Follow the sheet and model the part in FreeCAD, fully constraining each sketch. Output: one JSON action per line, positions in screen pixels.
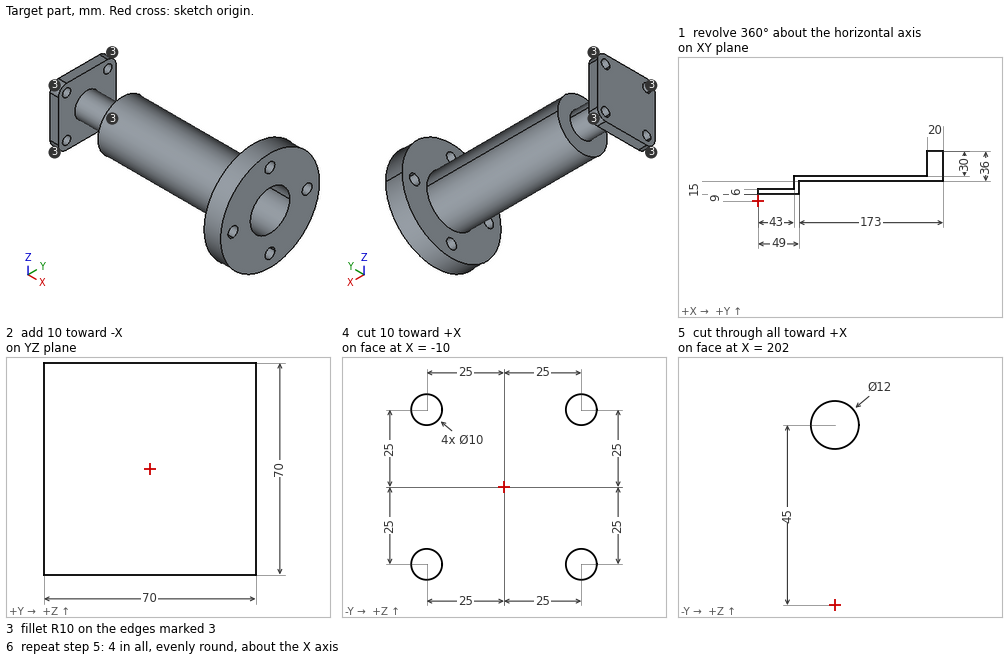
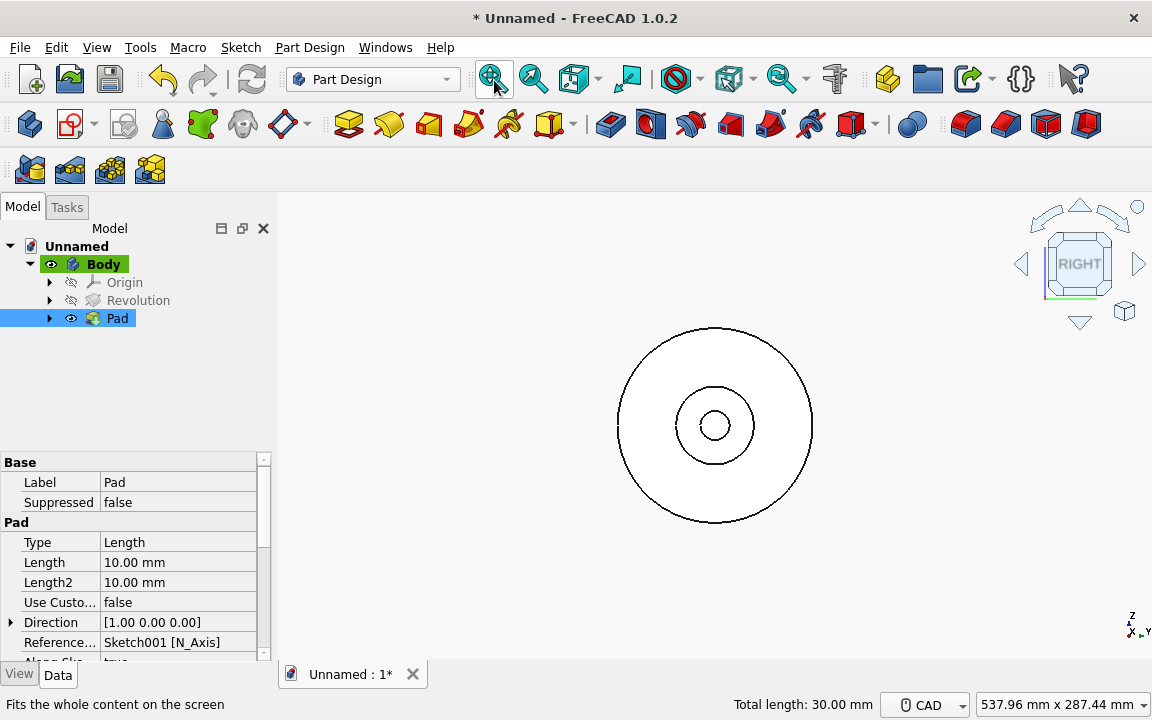
{"action": "left_click", "coordinate": [494, 80]}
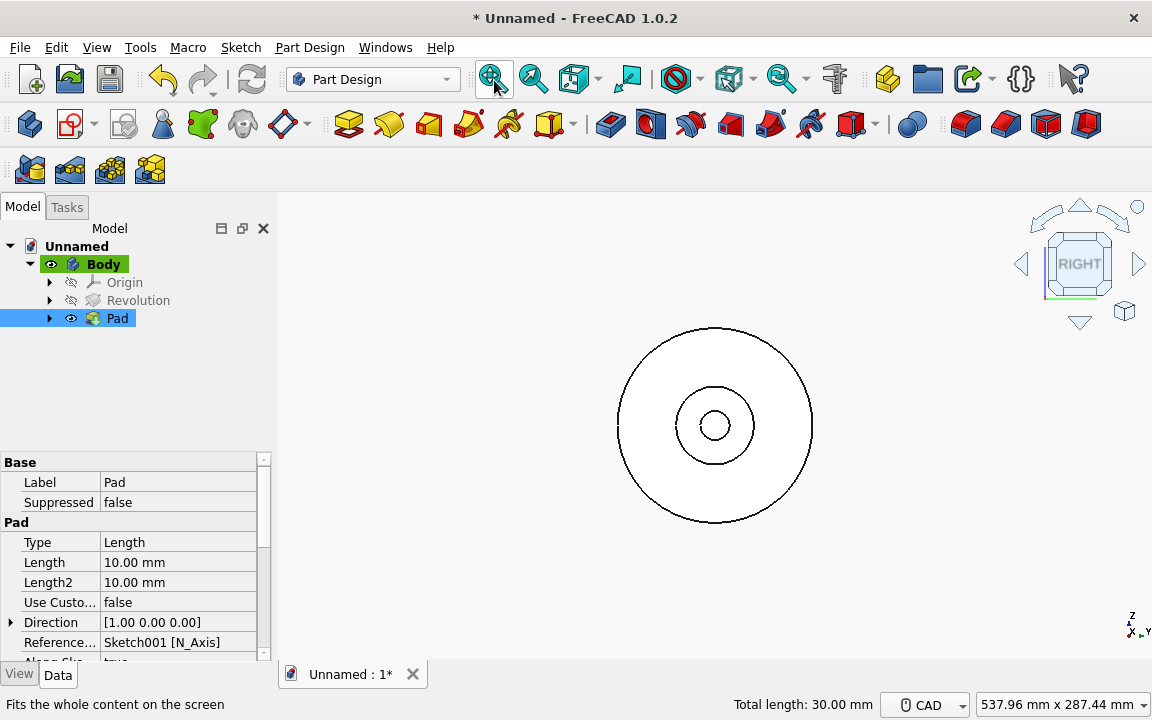
{"action": "scroll", "coordinate": [772, 481], "scroll_direction": "up", "scroll_amount": 5}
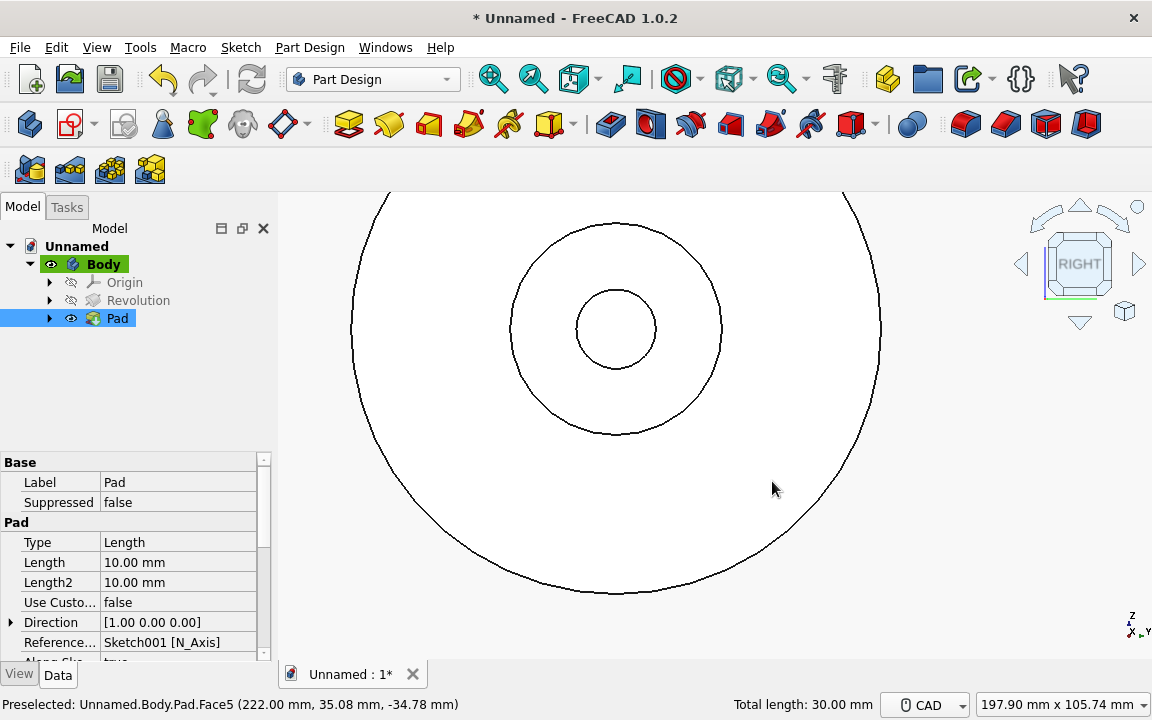
{"action": "left_click", "coordinate": [494, 80]}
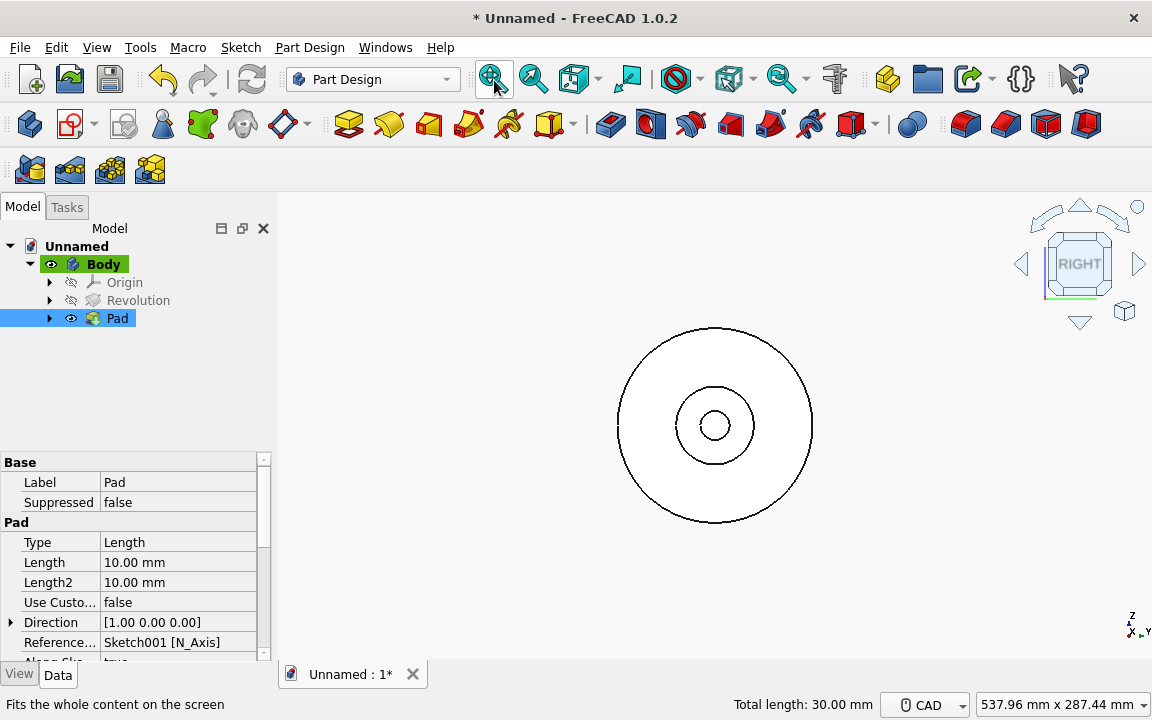
{"action": "key", "text": "5"}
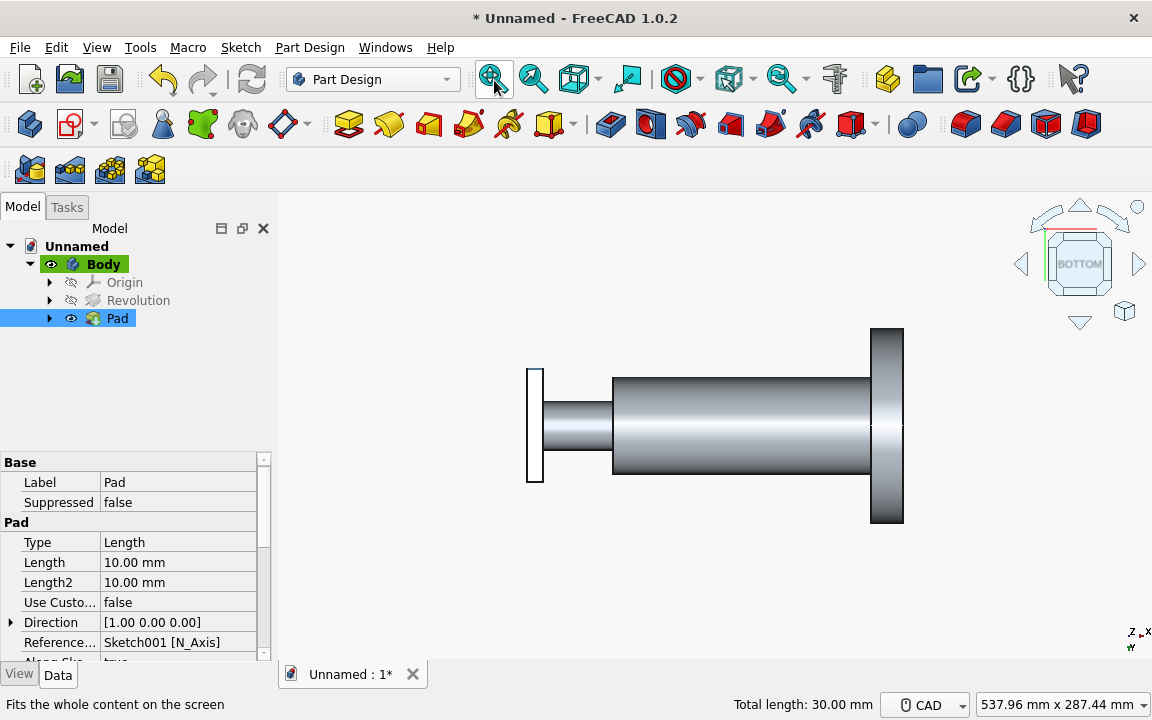
{"action": "key", "text": "v f"}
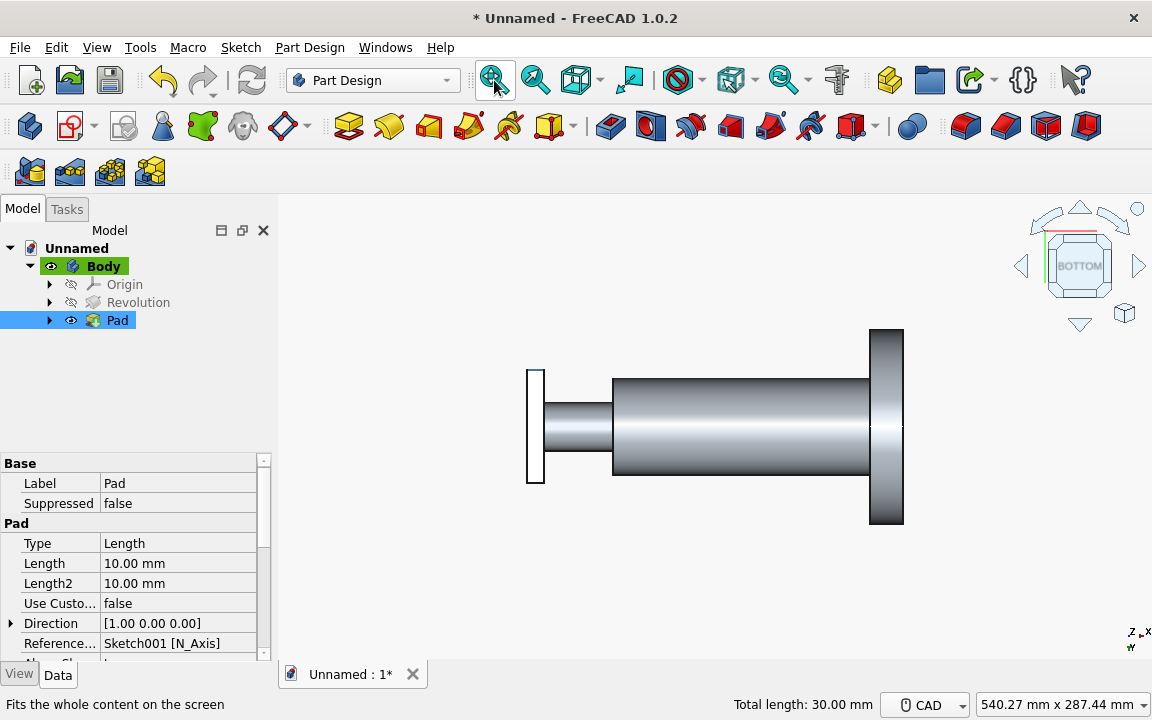
{"action": "left_click", "coordinate": [535, 482], "text": "ctrl"}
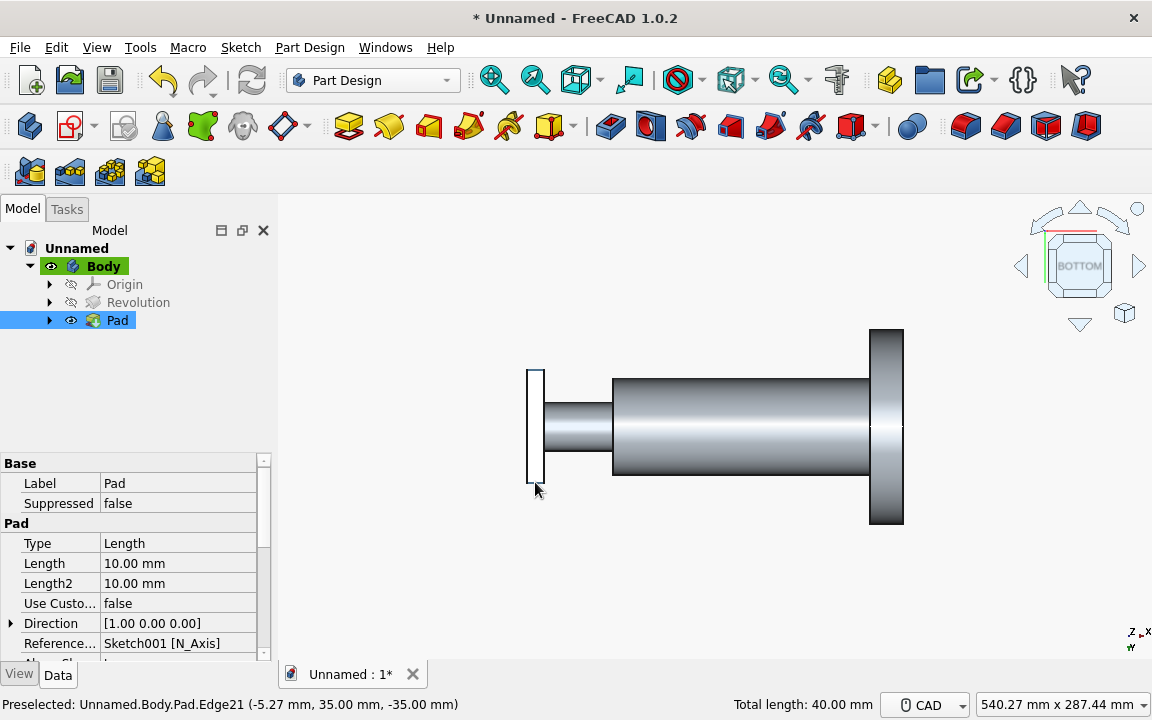
{"action": "left_click", "coordinate": [966, 126]}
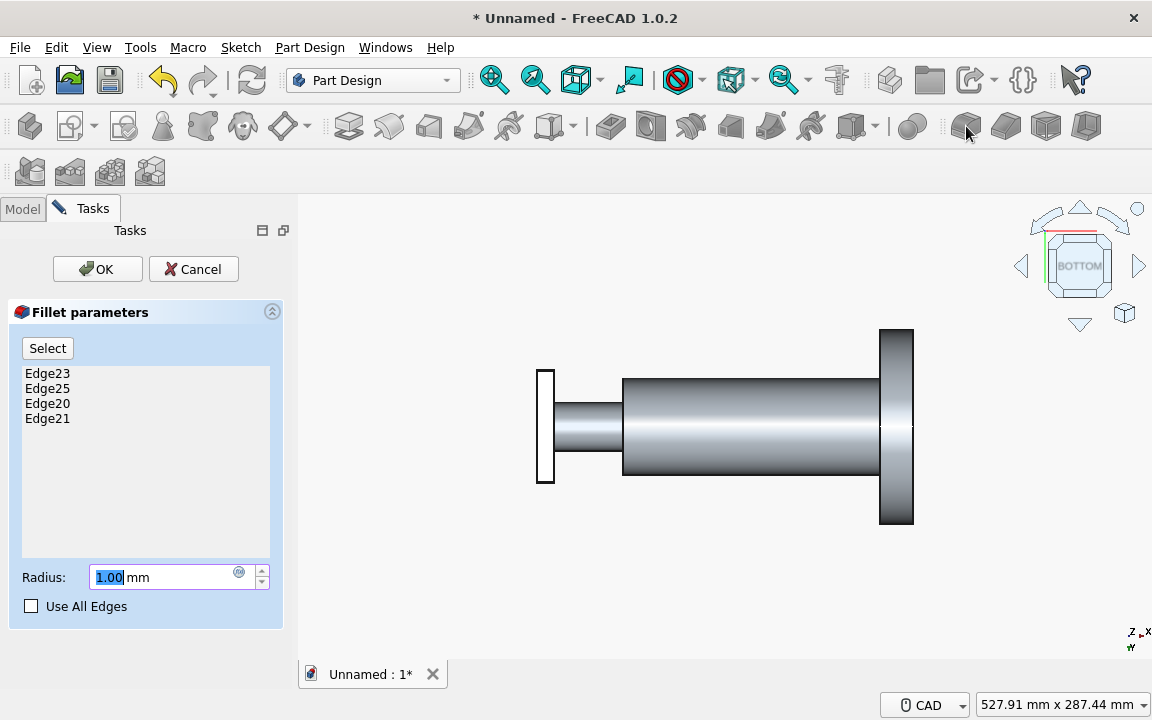
{"action": "type", "text": "10"}
{"action": "key", "text": "Tab"}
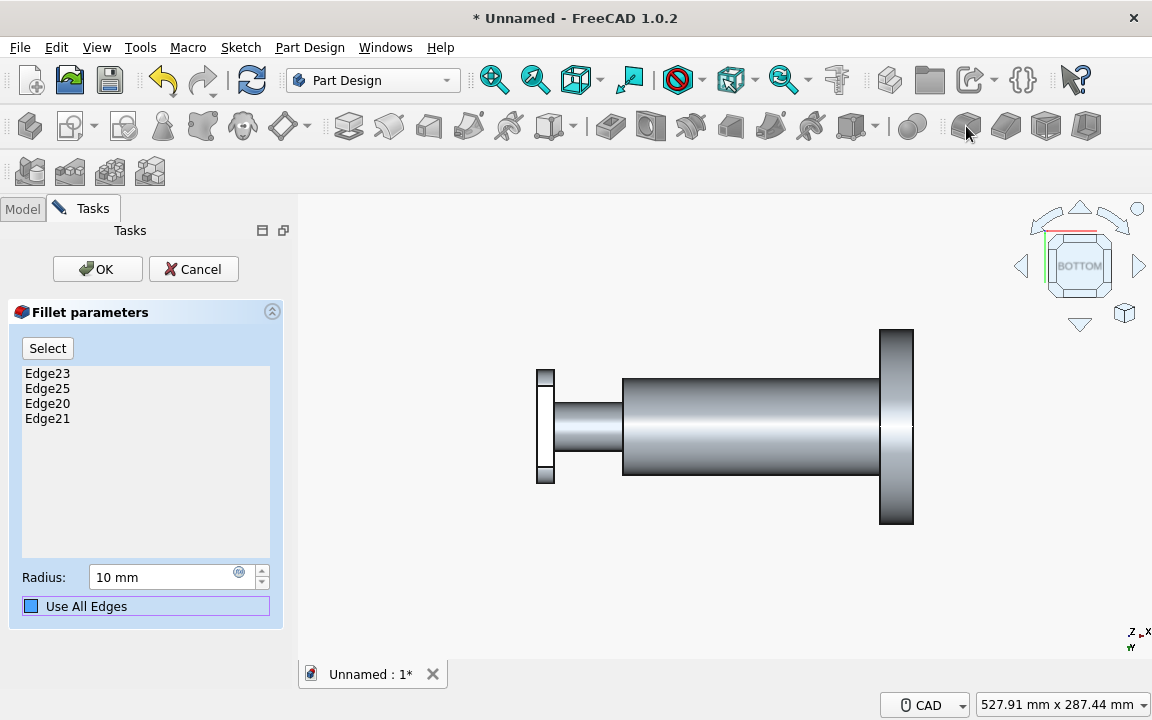
{"action": "left_click", "coordinate": [98, 269]}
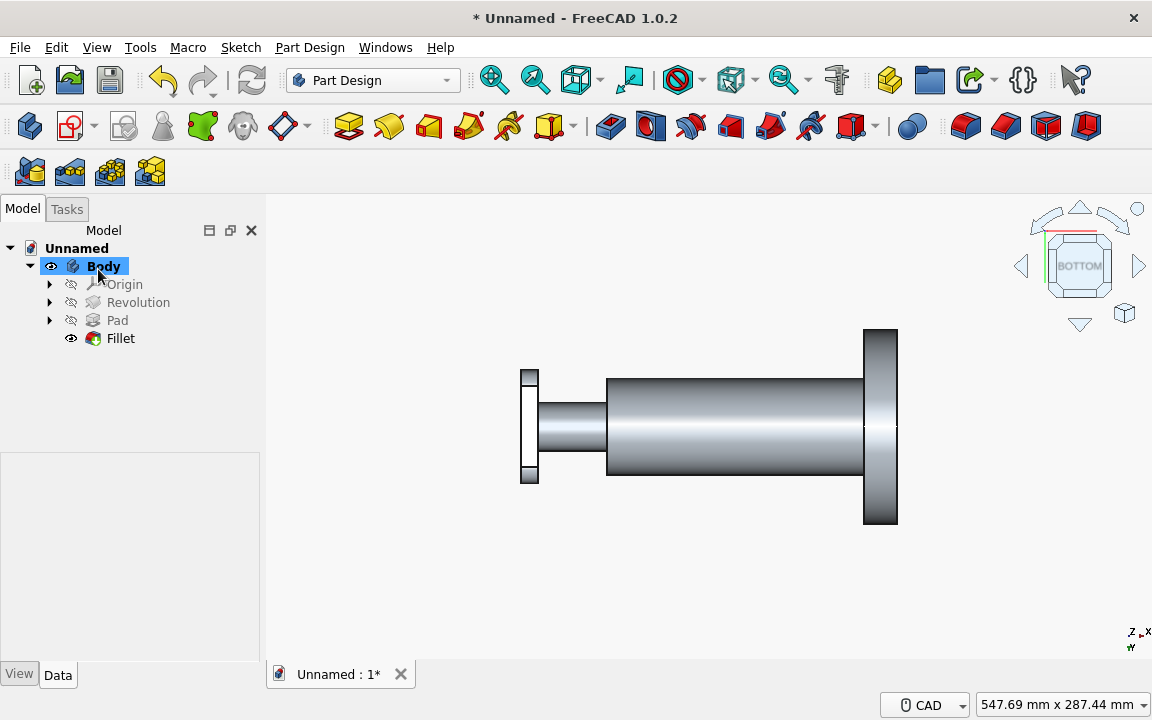
{"action": "left_click", "coordinate": [496, 80]}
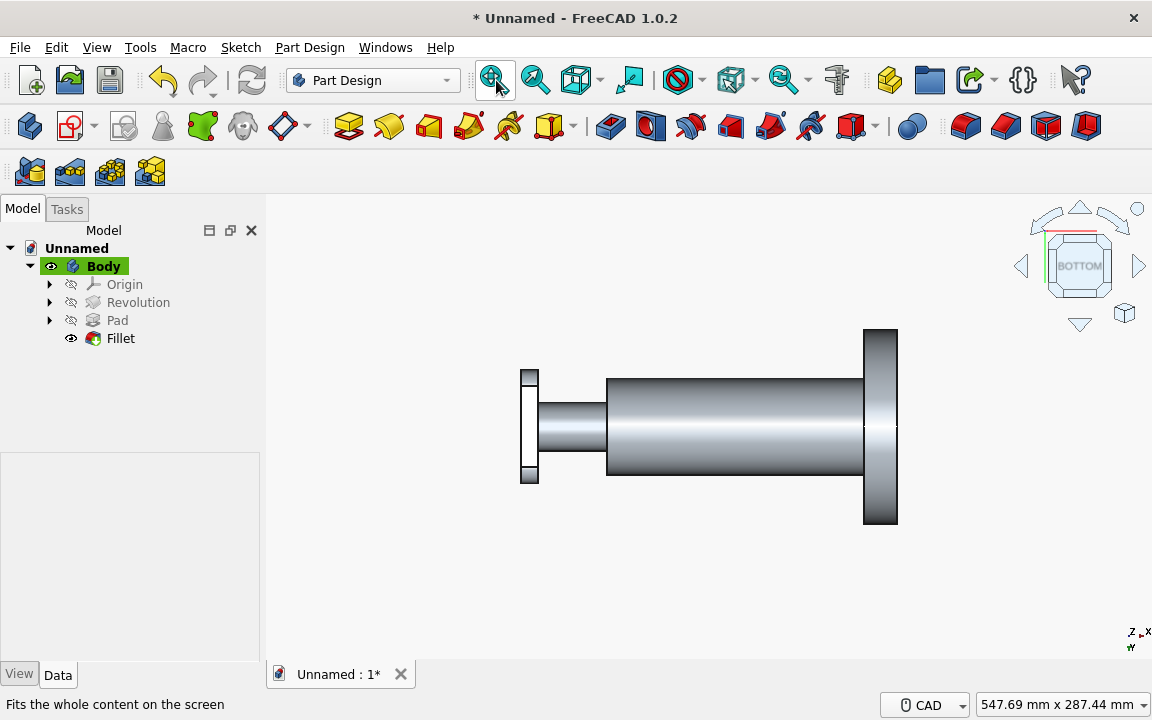
{"action": "key", "text": "6"}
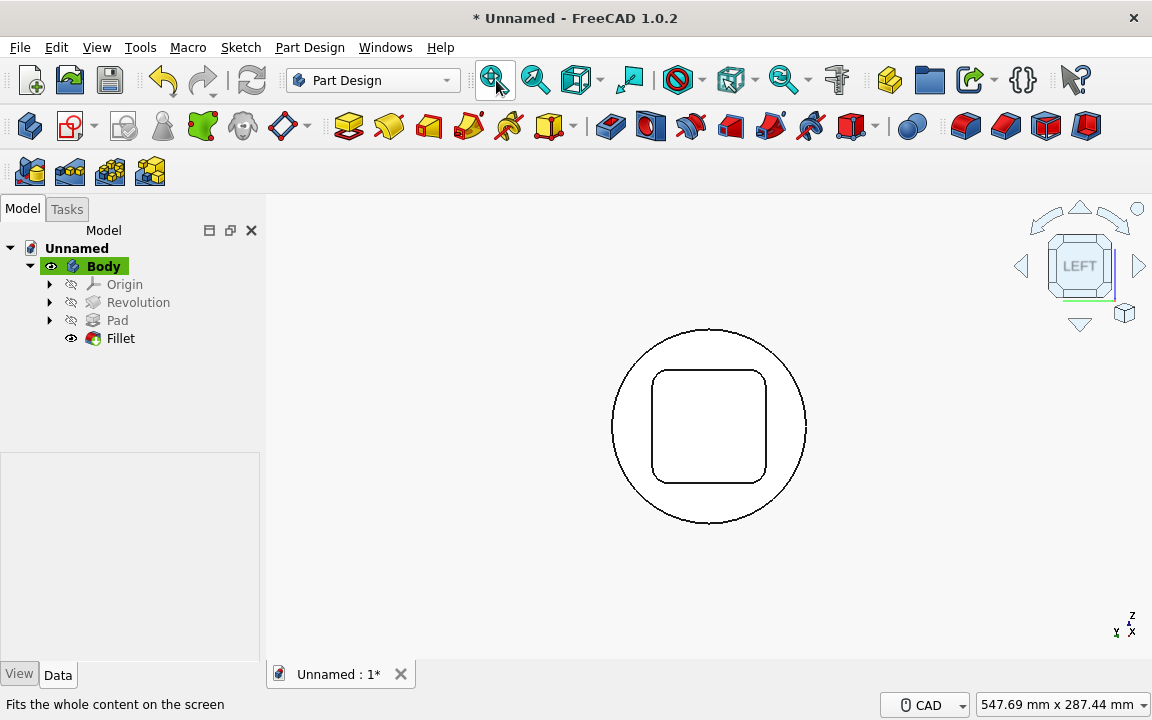
{"action": "left_click", "coordinate": [496, 80]}